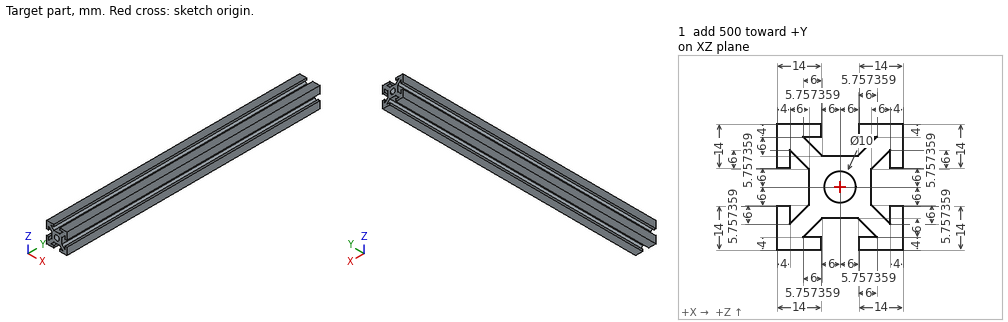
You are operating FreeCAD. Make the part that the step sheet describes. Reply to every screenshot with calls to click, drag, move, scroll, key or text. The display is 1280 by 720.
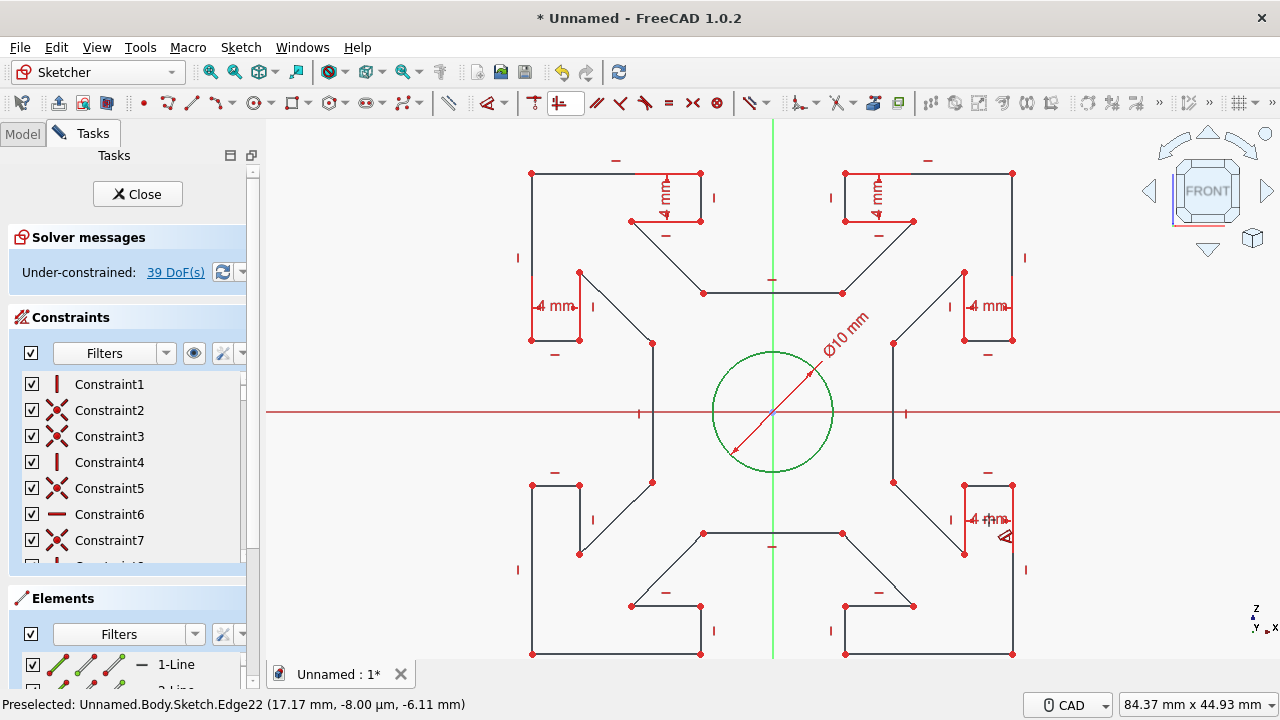
click(845, 621)
click(879, 624)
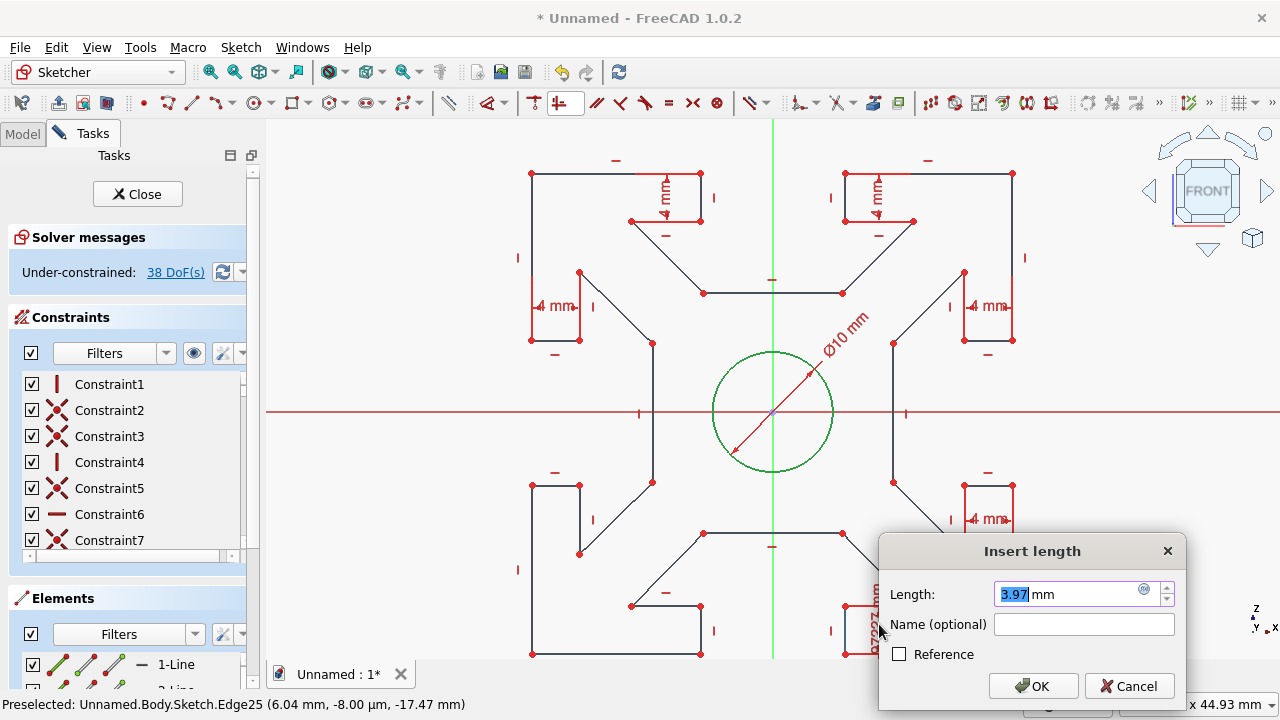
text(4)
key(Return)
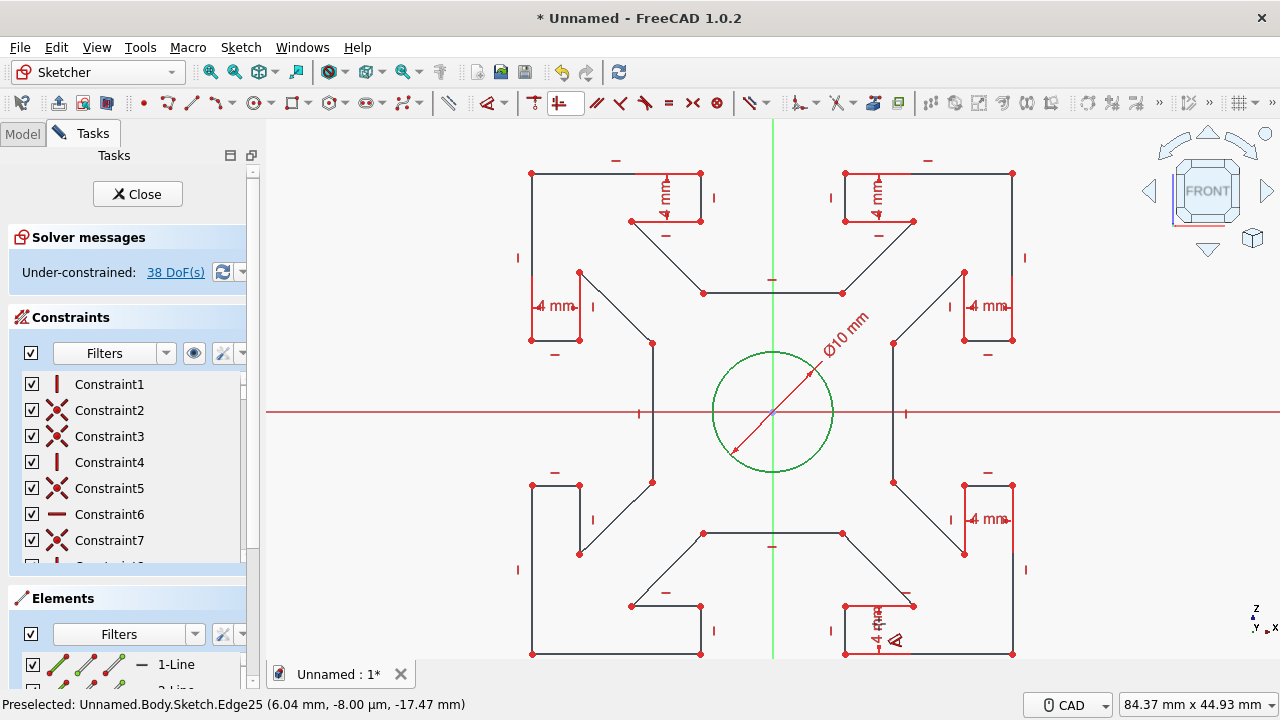
click(701, 621)
click(667, 624)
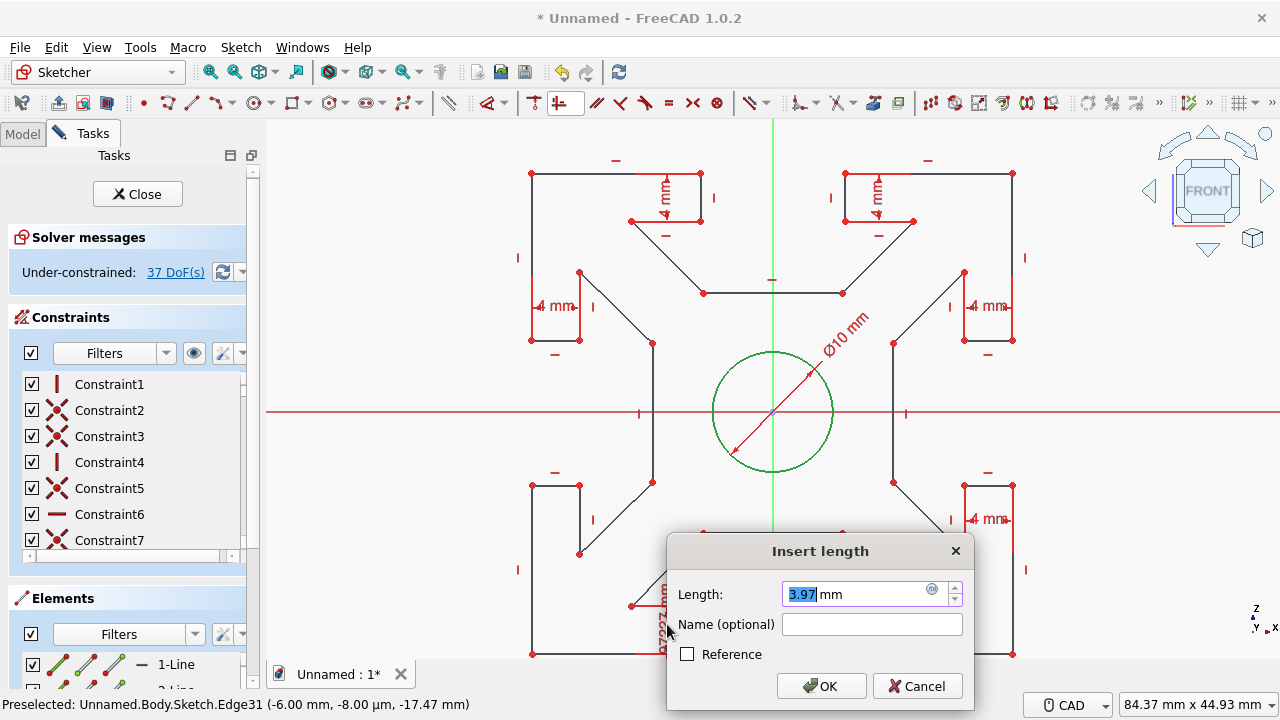
text(4)
key(Return)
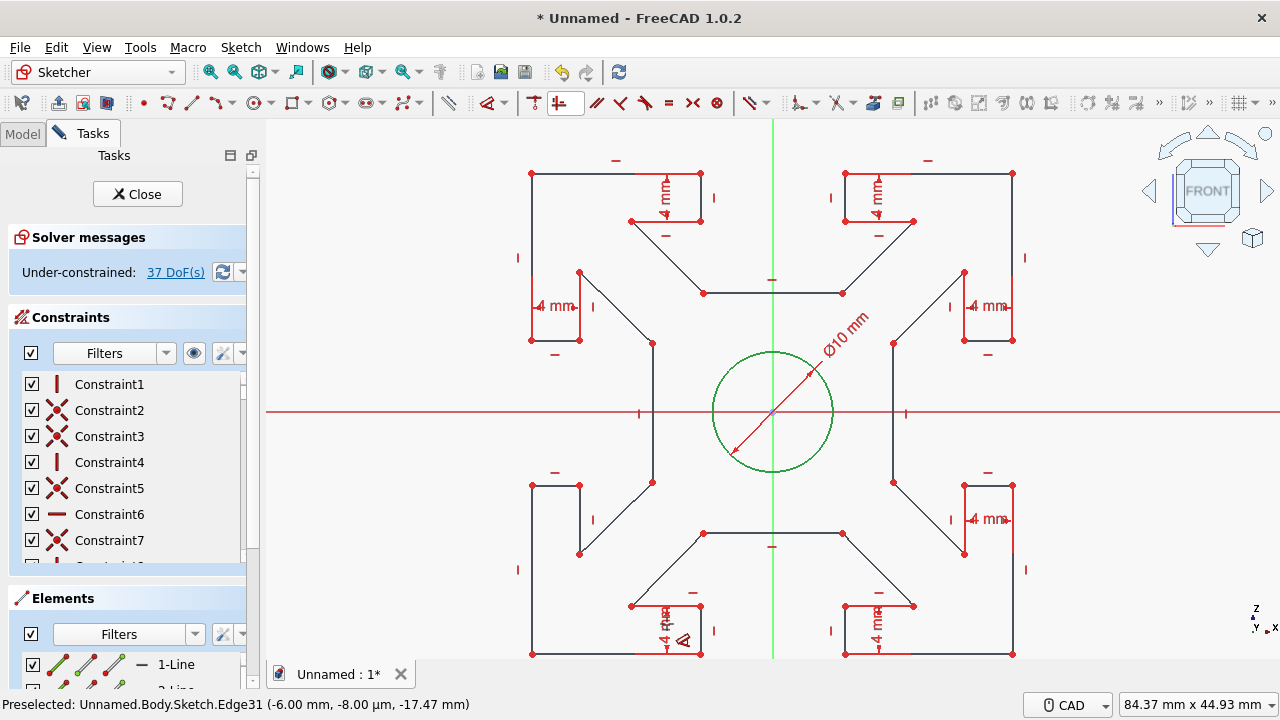
click(546, 486)
click(556, 520)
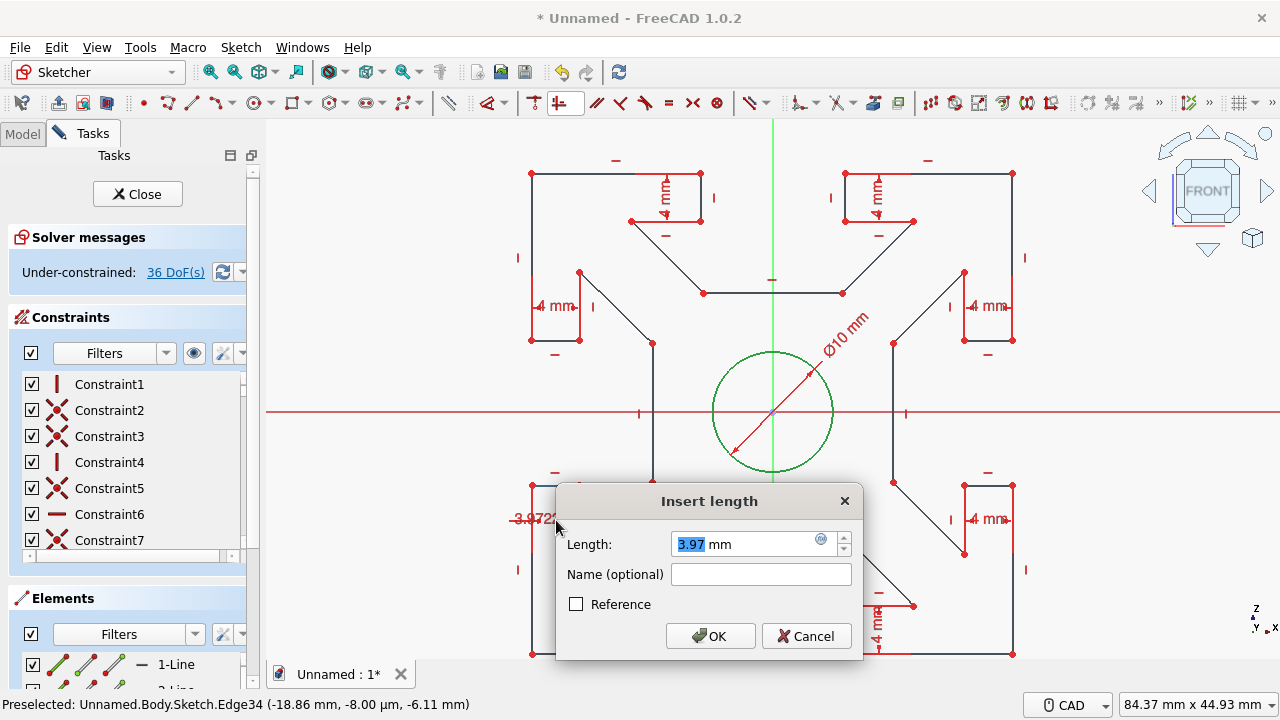
text(4)
key(Return)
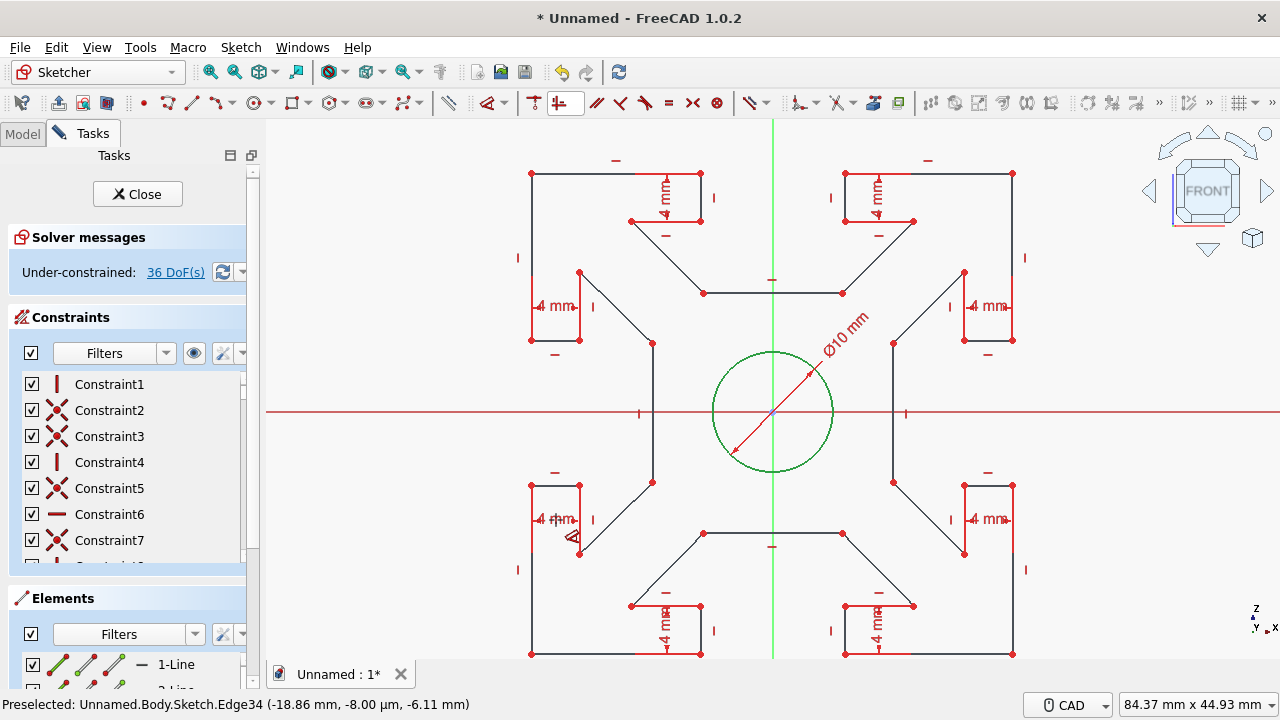
click(532, 291)
click(498, 257)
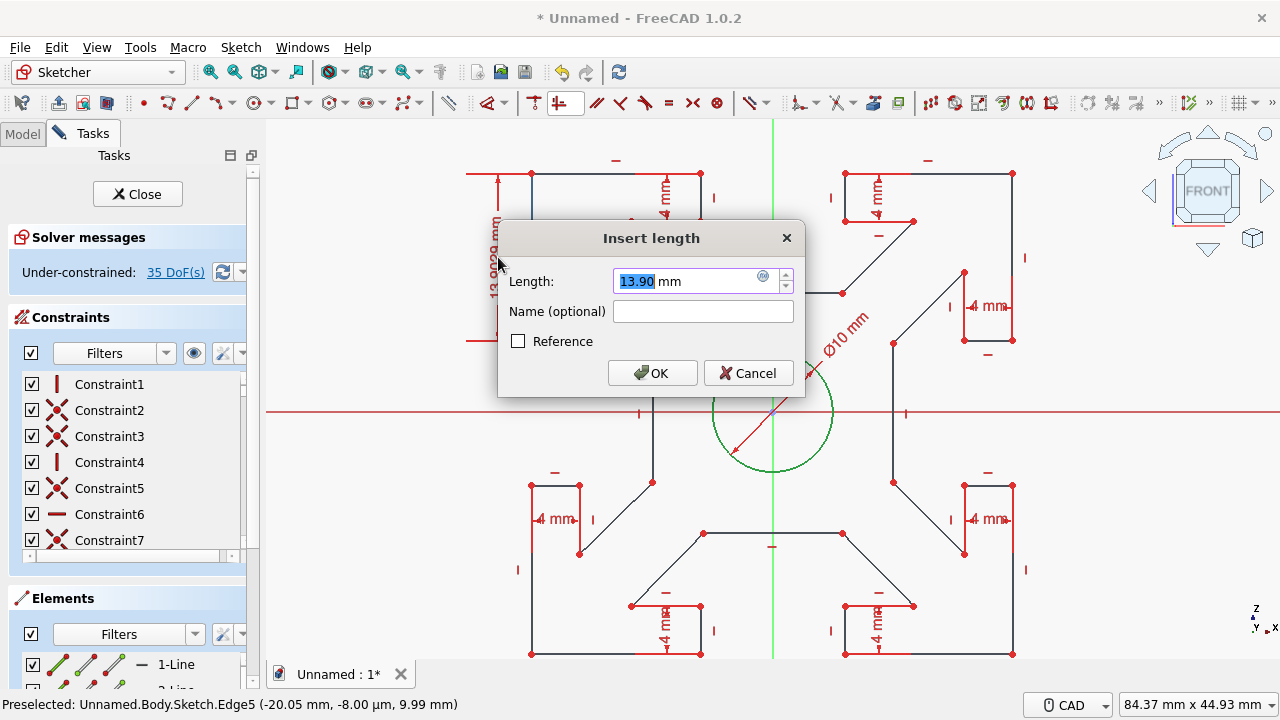
text(14)
key(Return)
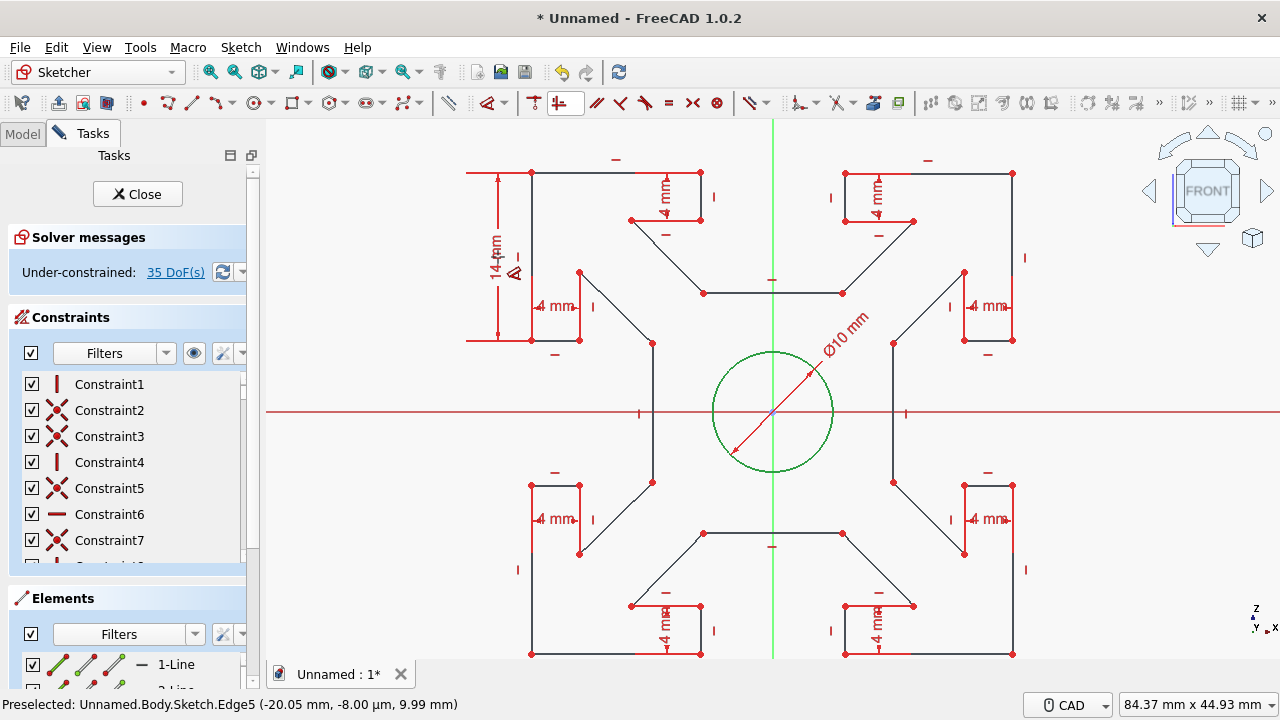
click(582, 173)
click(577, 207)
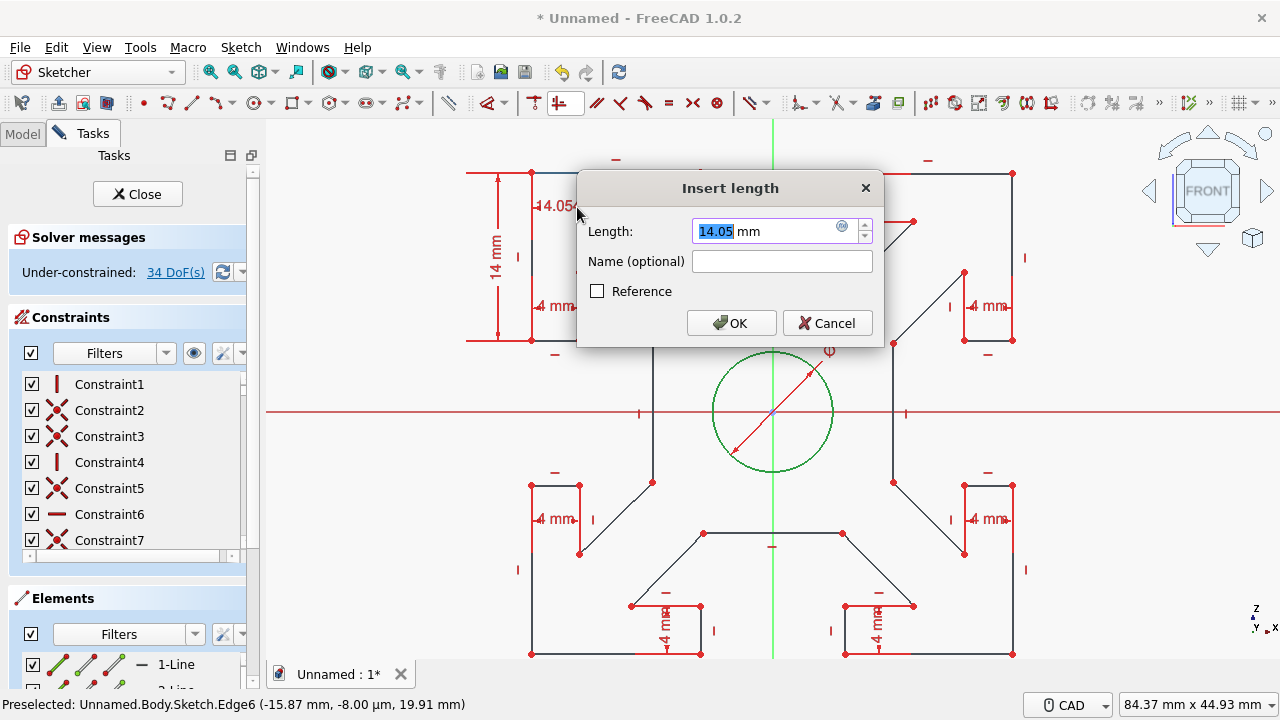
text(14)
key(Return)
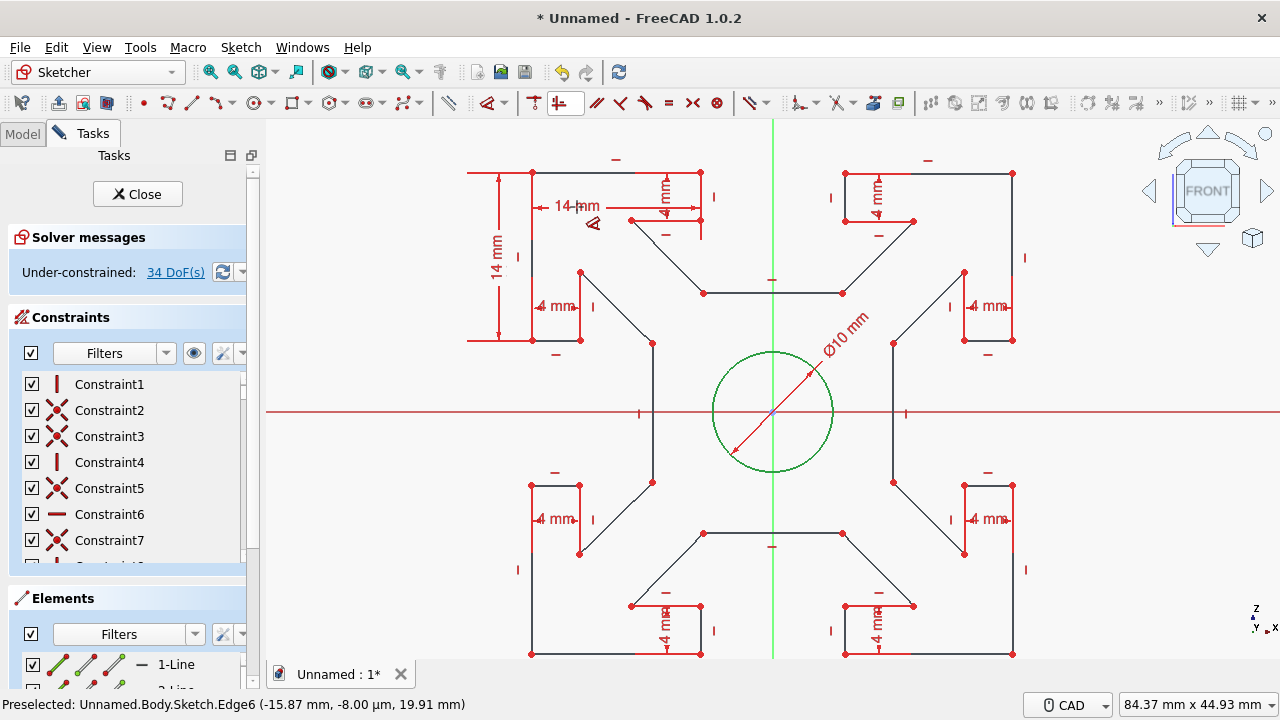
click(895, 174)
click(967, 208)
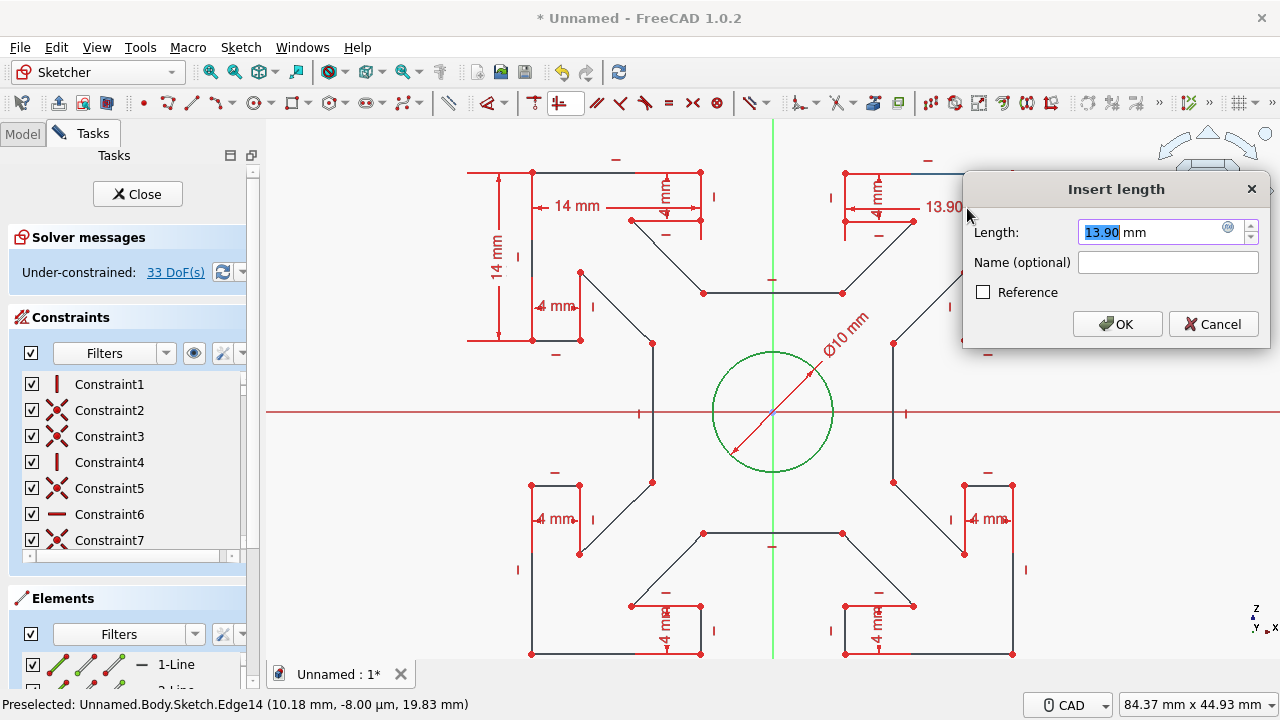
text(14)
key(Return)